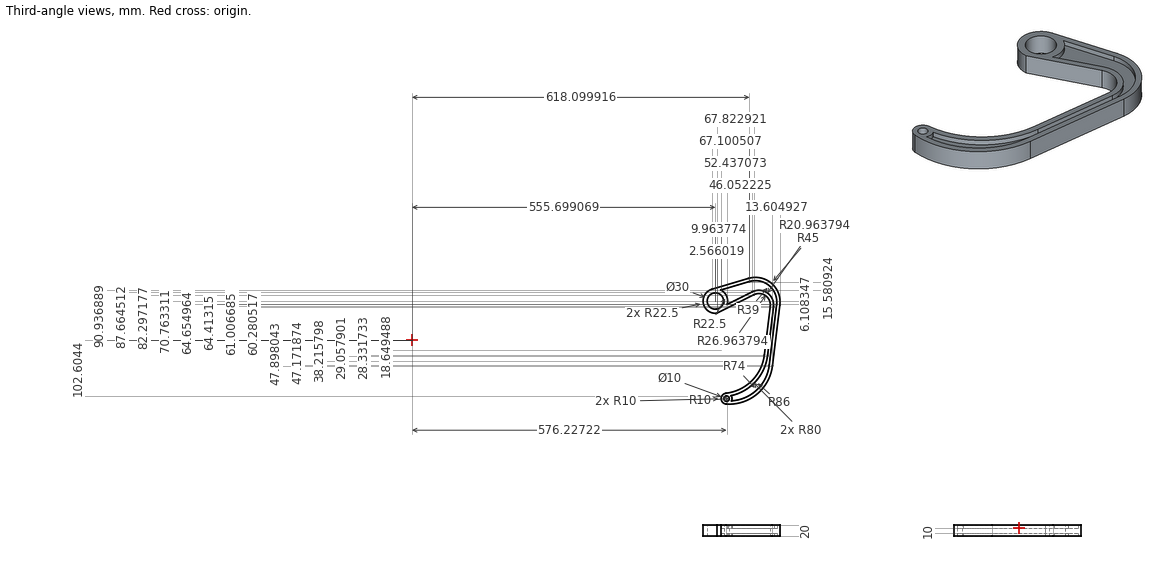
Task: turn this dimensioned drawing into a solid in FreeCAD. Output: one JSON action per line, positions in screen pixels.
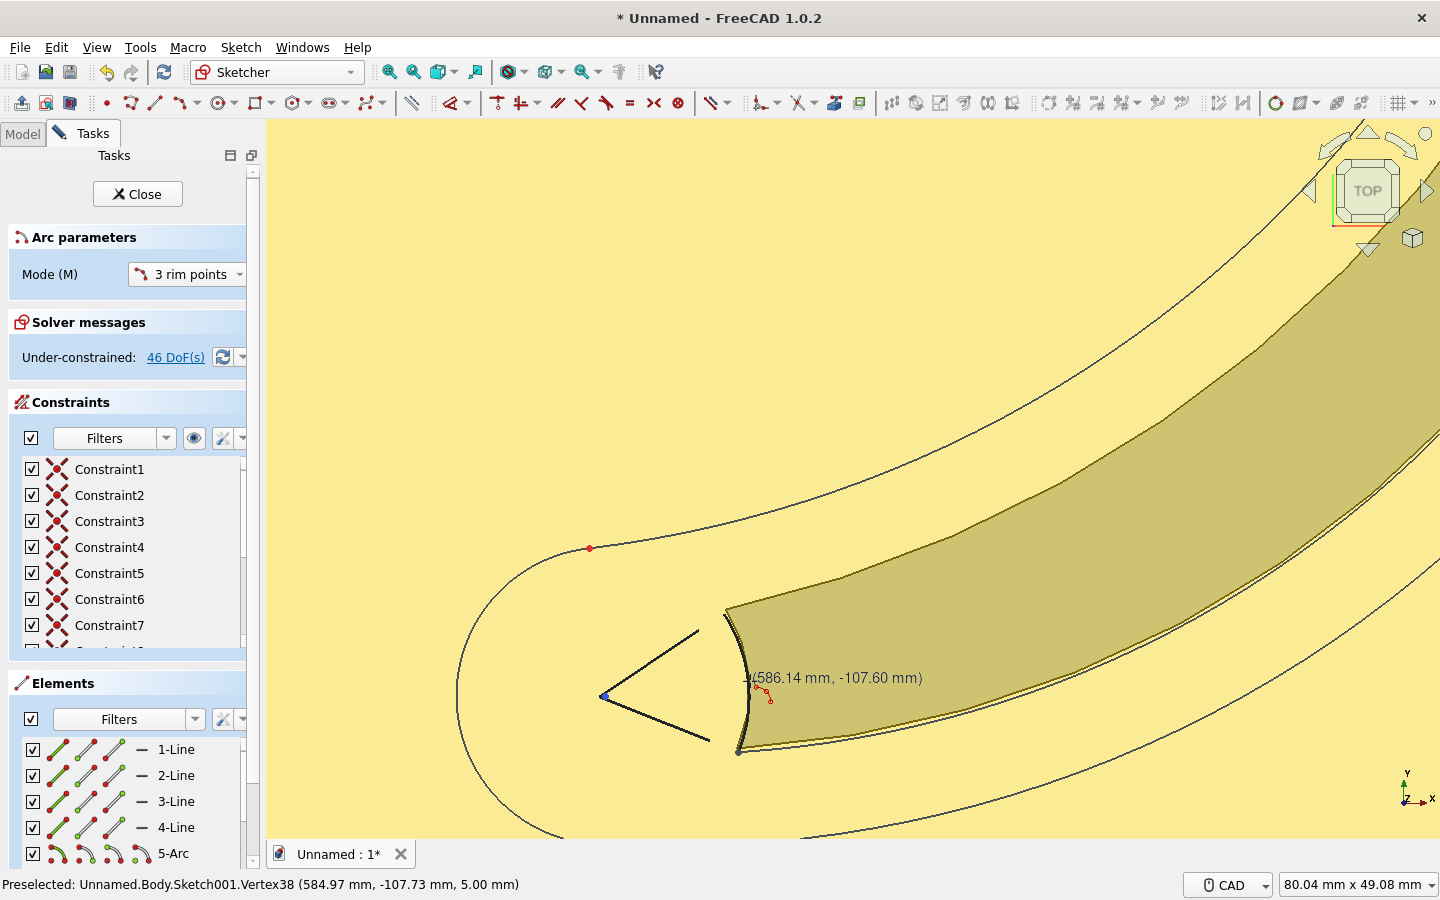
{"action": "left_click", "coordinate": [749, 678]}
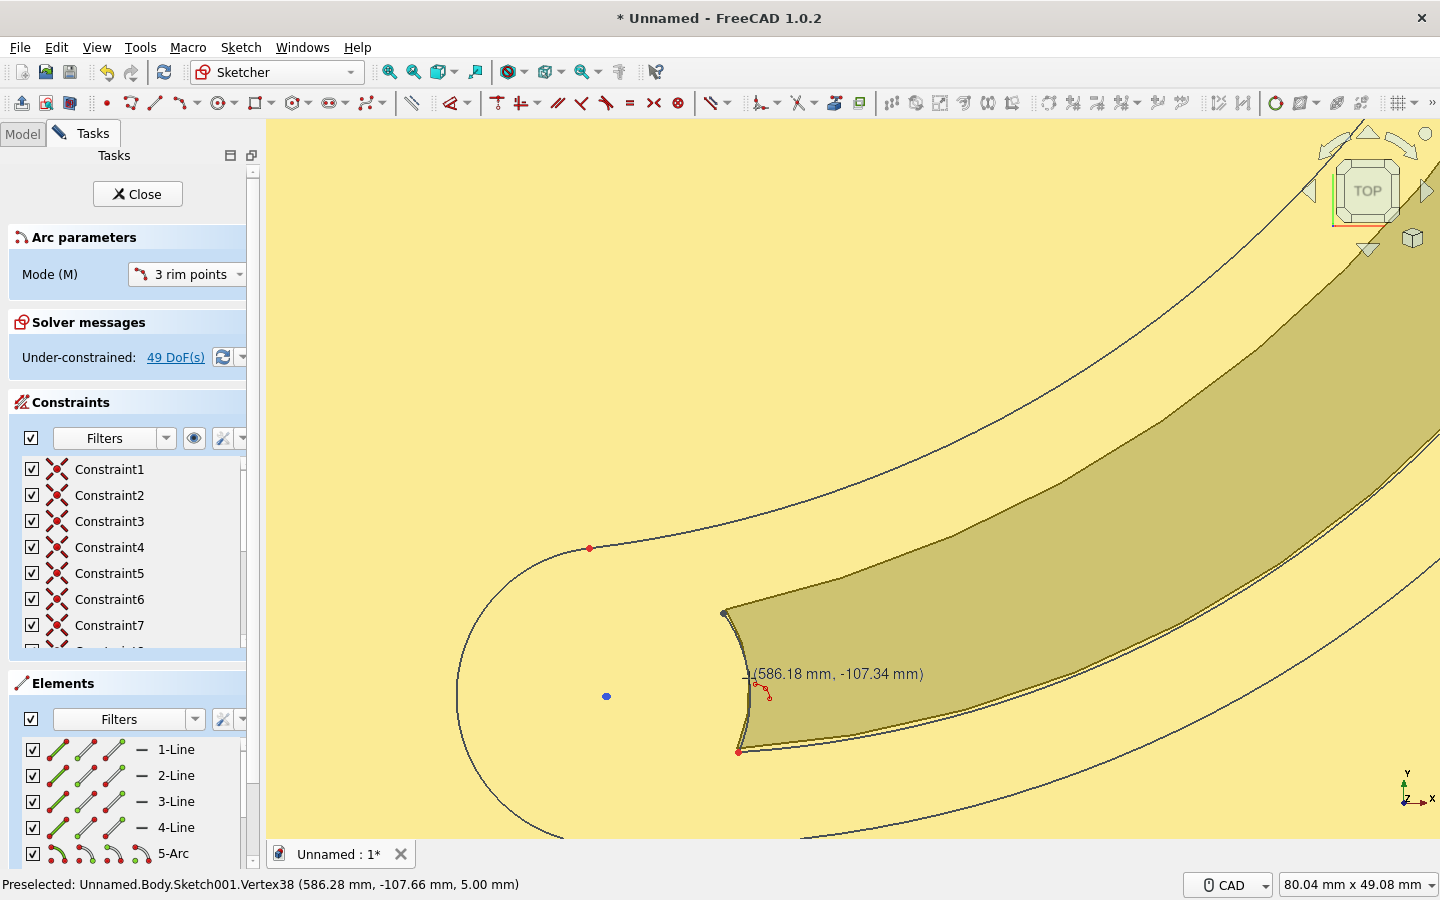
{"action": "scroll", "coordinate": [750, 688], "scroll_direction": "down", "scroll_amount": 10}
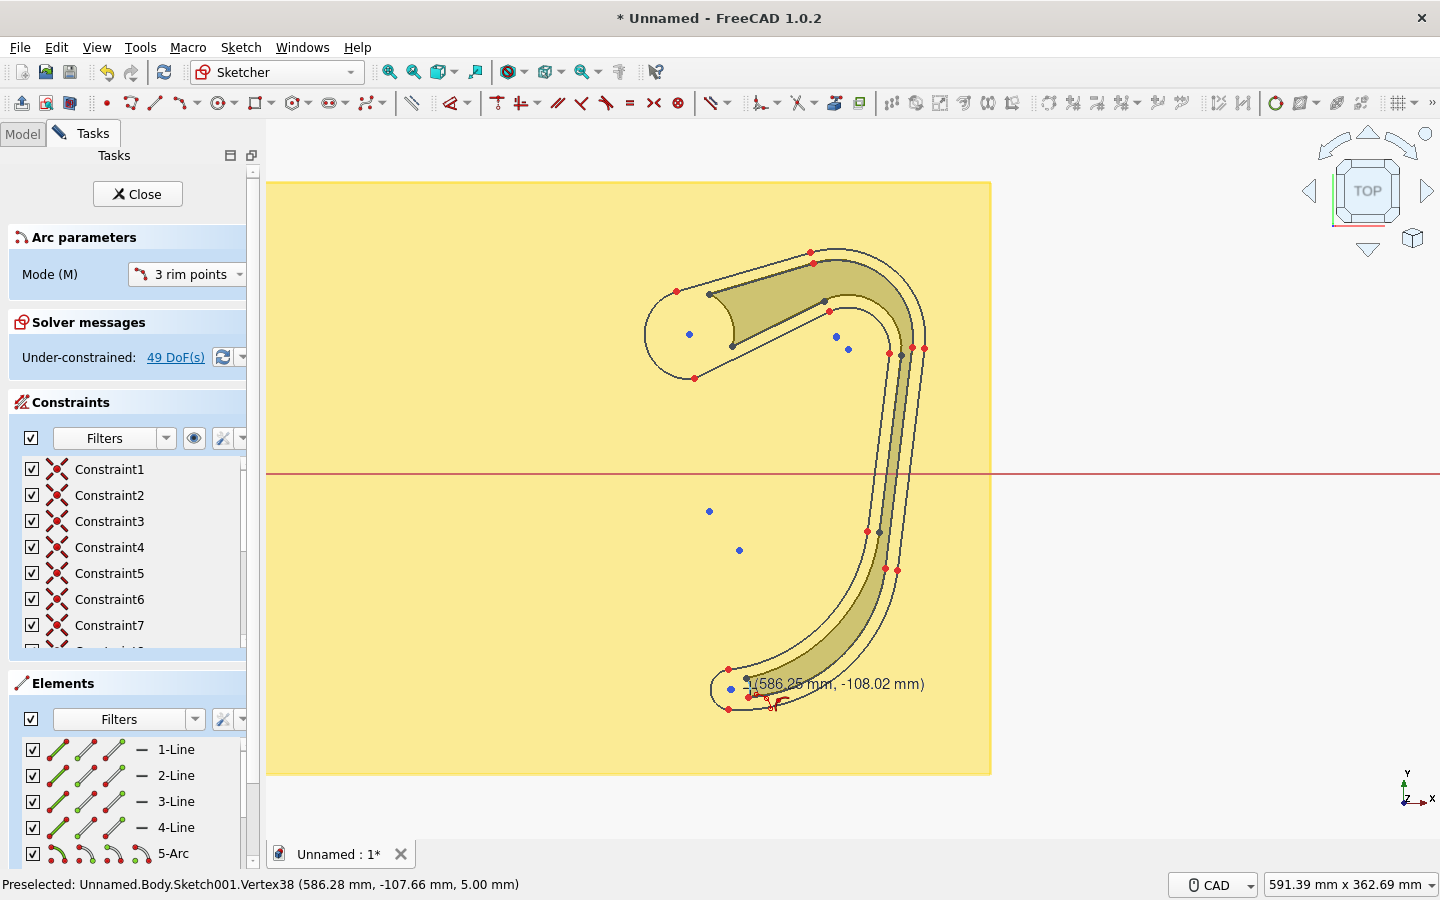
{"action": "scroll", "coordinate": [747, 678], "scroll_direction": "up", "scroll_amount": 2}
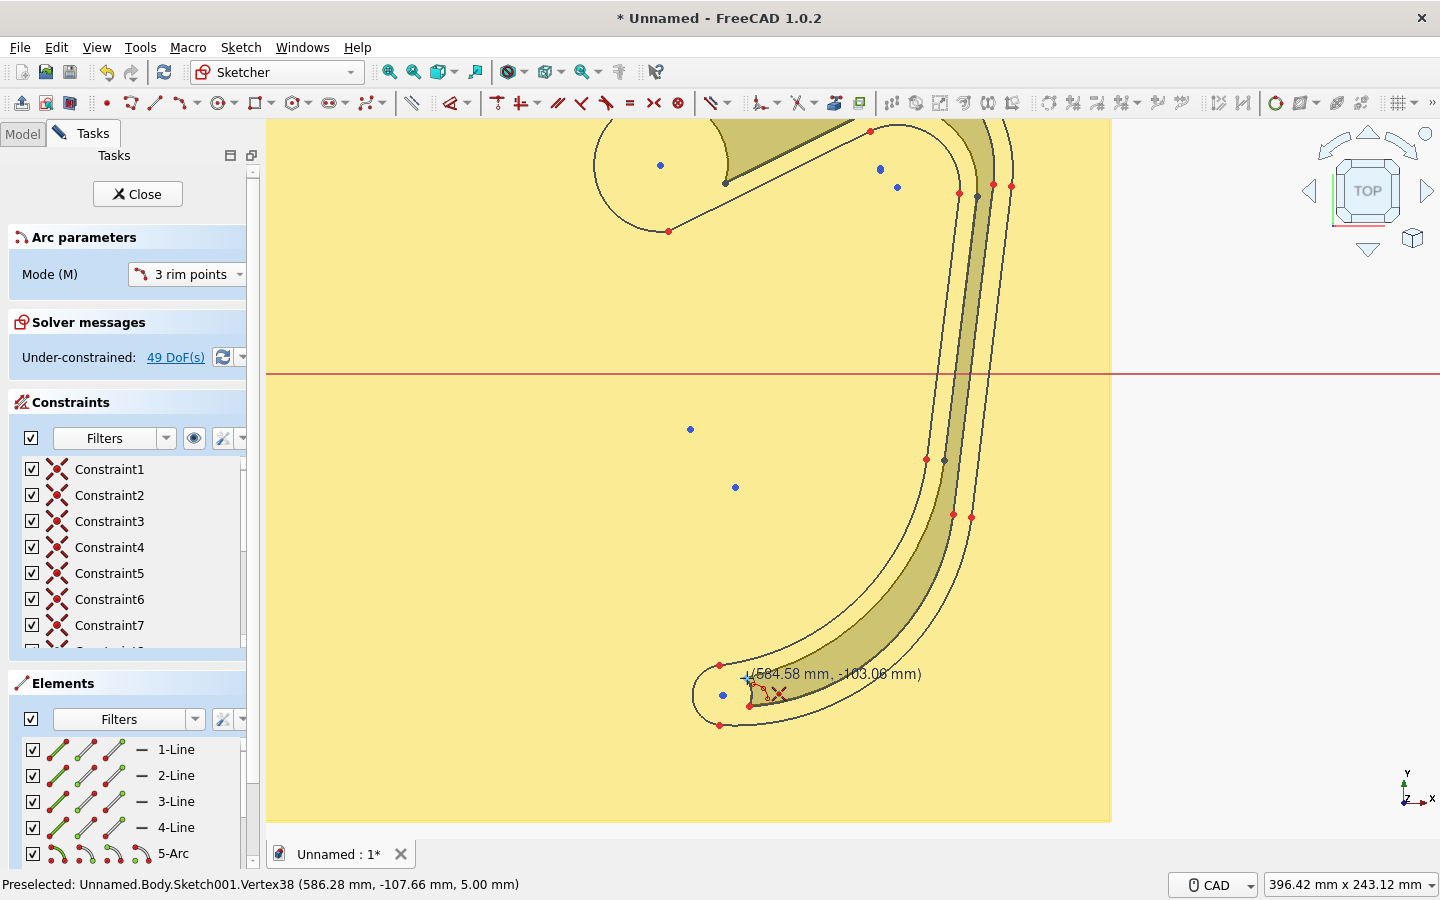
{"action": "left_click", "coordinate": [746, 679]}
{"action": "left_click", "coordinate": [944, 461]}
{"action": "left_click", "coordinate": [900, 576]}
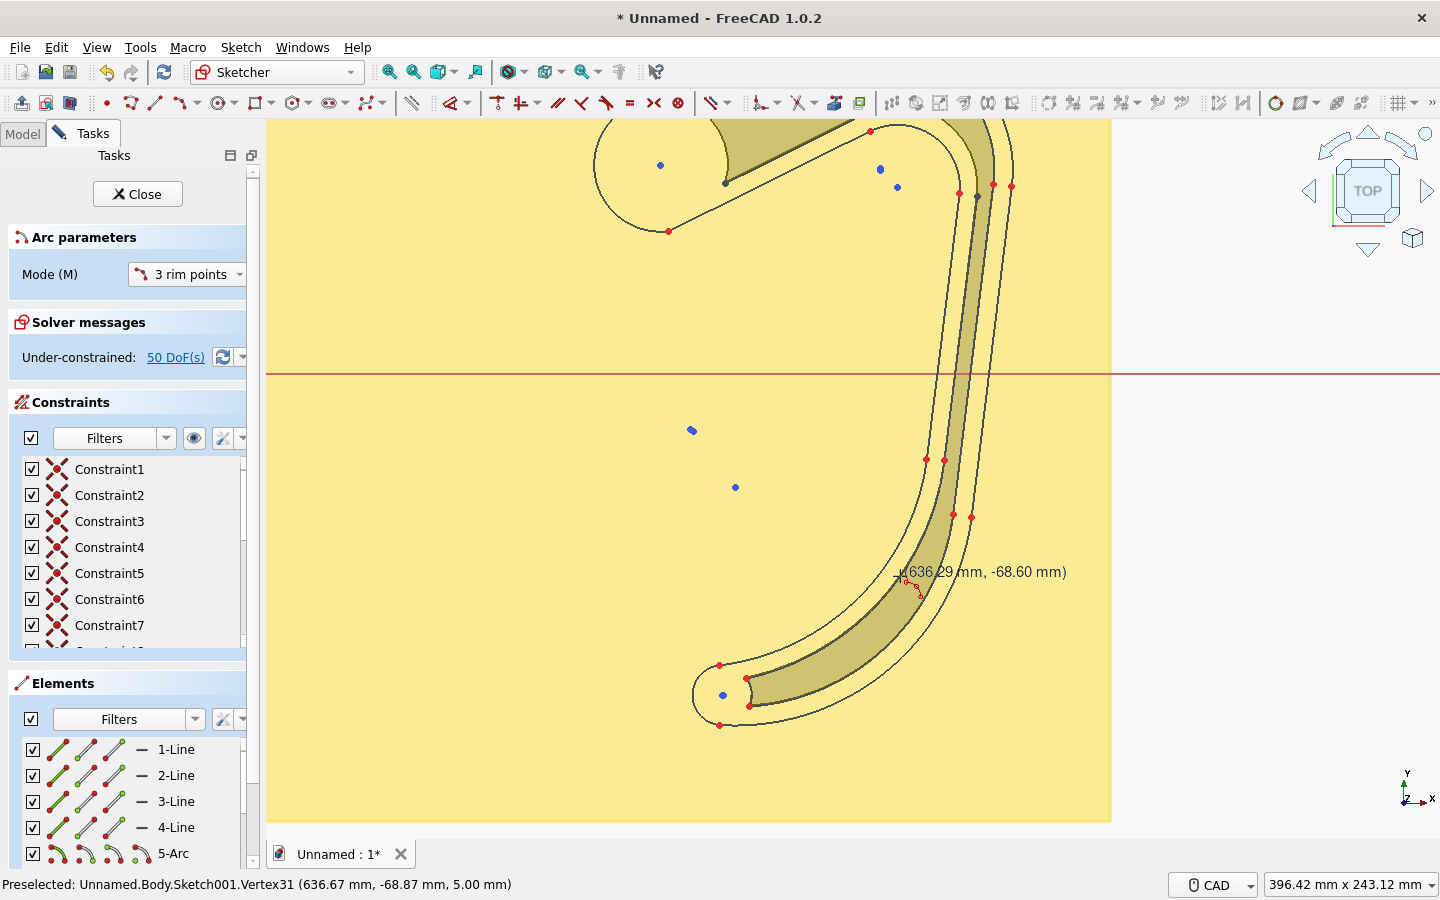
{"action": "left_click", "coordinate": [977, 197]}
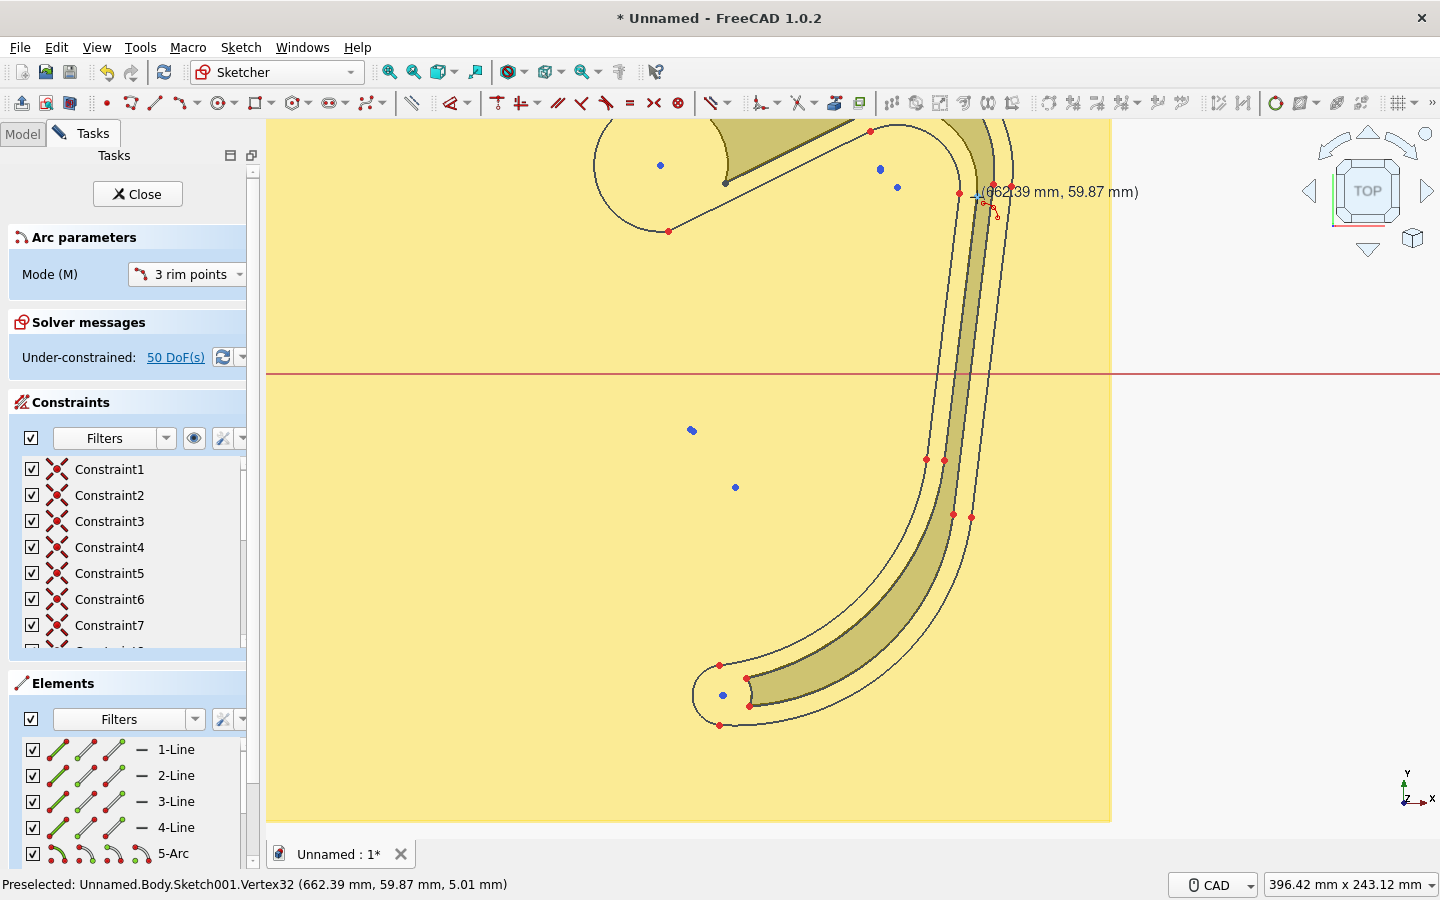
{"action": "scroll", "coordinate": [746, 675], "scroll_direction": "down", "scroll_amount": 2}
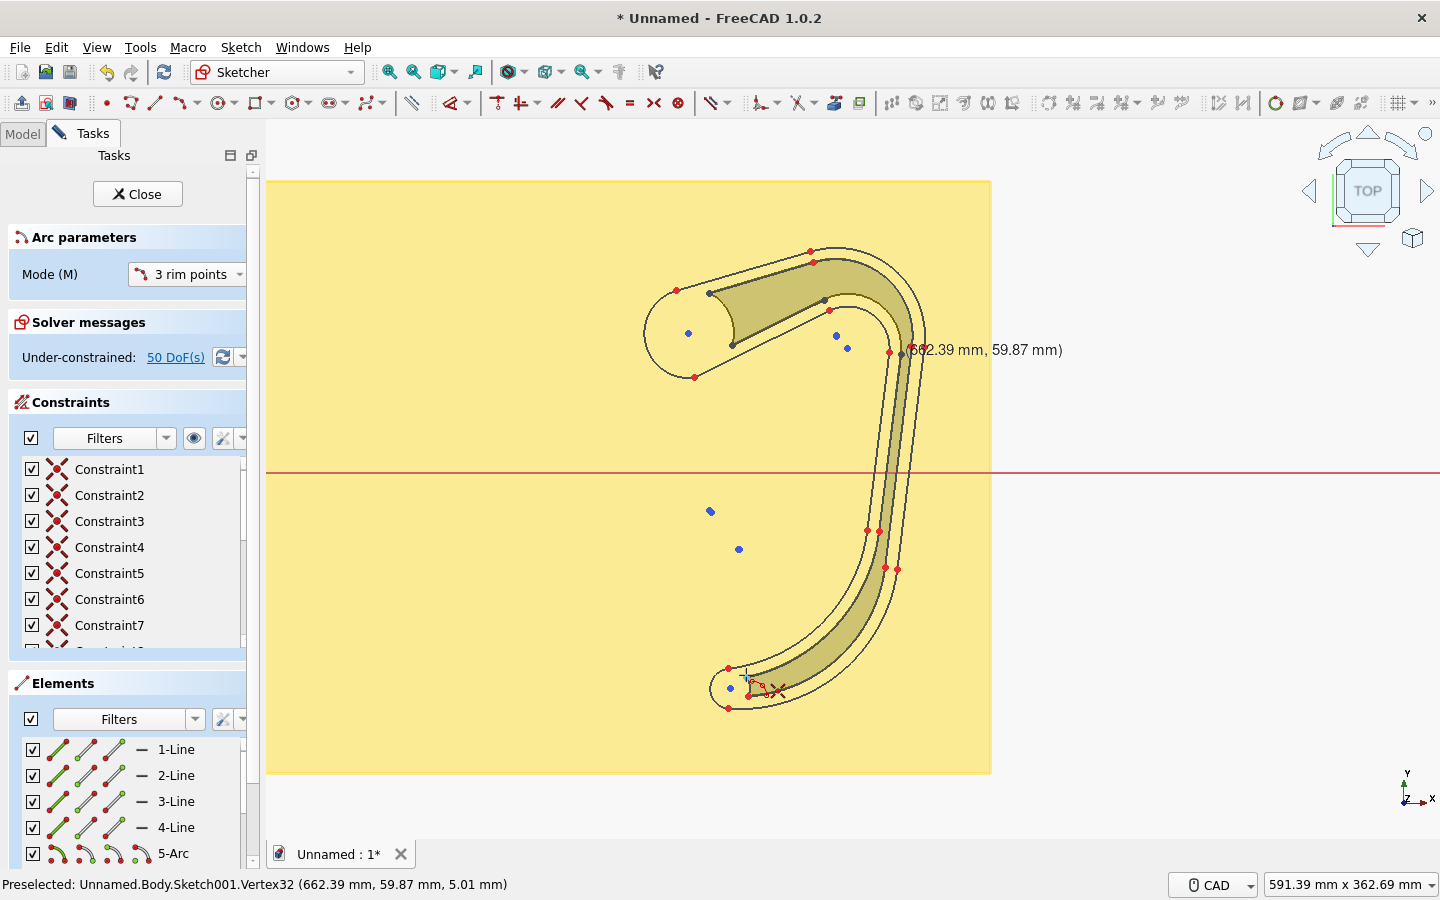
{"action": "scroll", "coordinate": [824, 299], "scroll_direction": "up", "scroll_amount": 2}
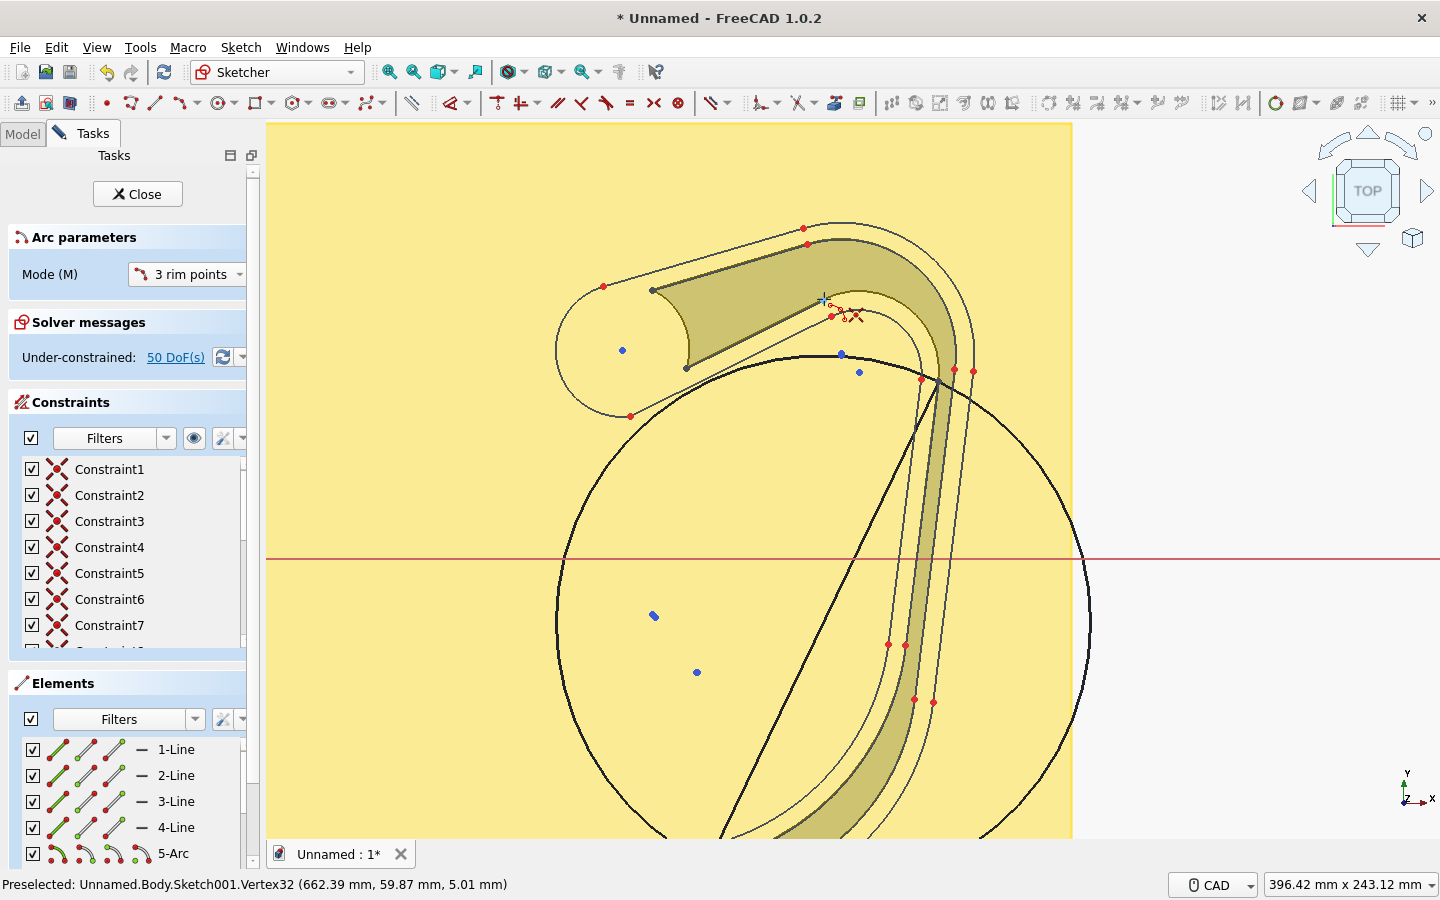
{"action": "left_click", "coordinate": [824, 301]}
{"action": "left_click", "coordinate": [890, 297]}